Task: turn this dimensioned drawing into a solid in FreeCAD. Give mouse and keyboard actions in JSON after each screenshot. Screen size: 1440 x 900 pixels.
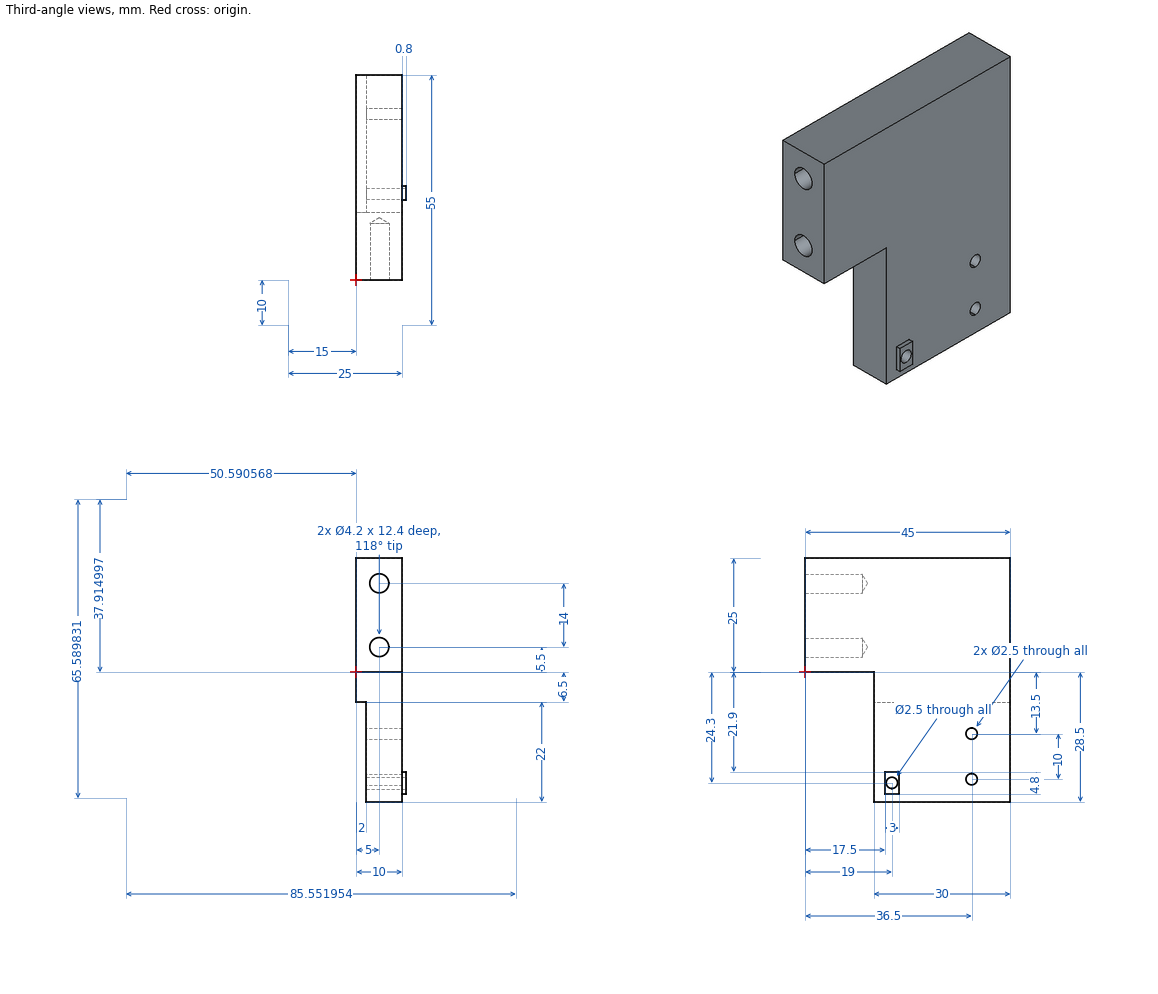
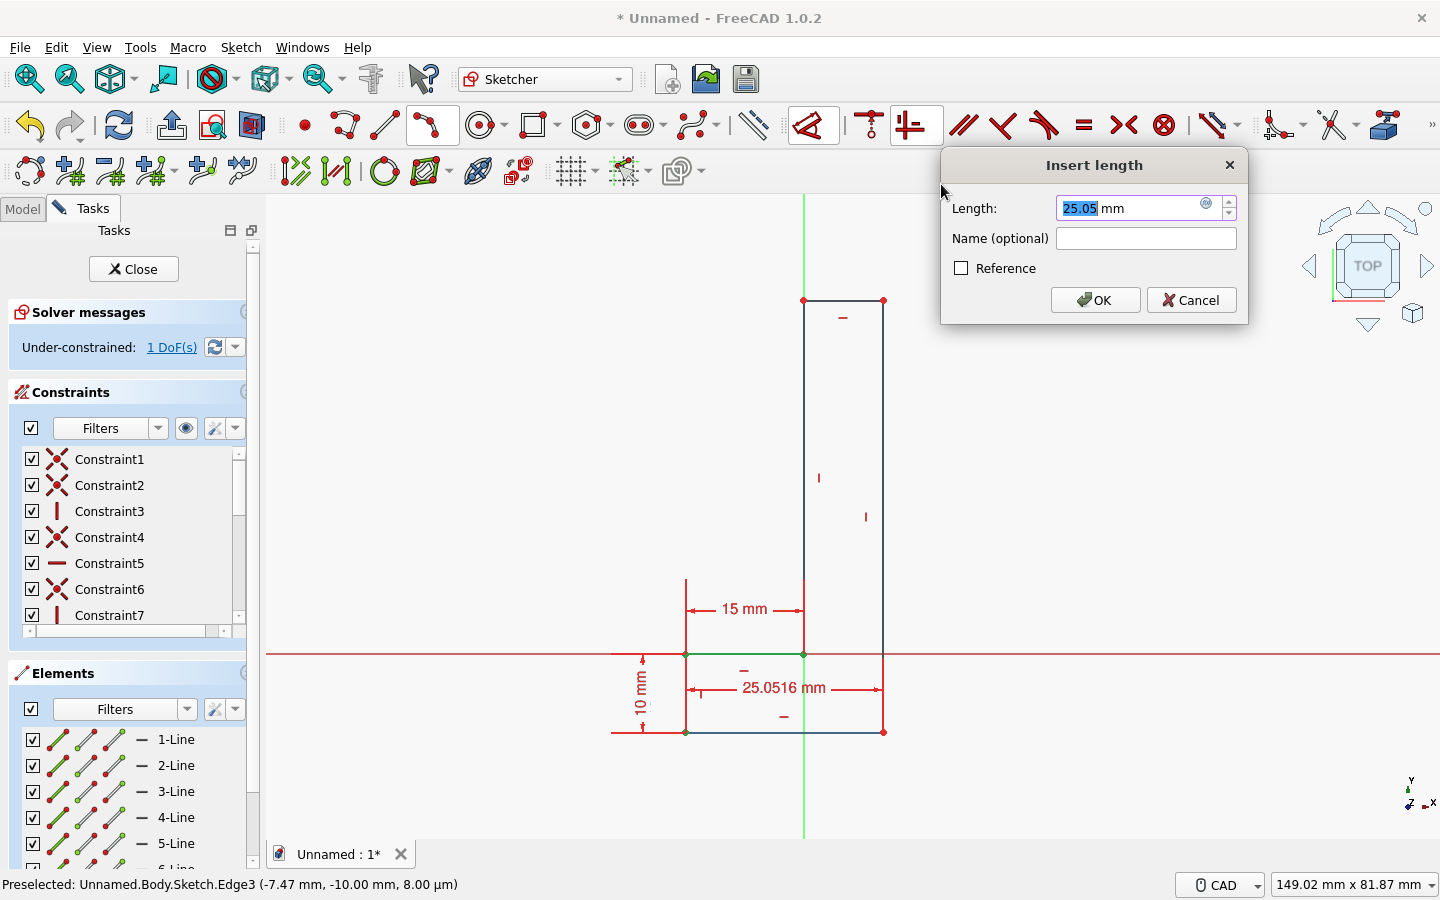
{"action": "type", "text": "25"}
{"action": "key", "text": "Return"}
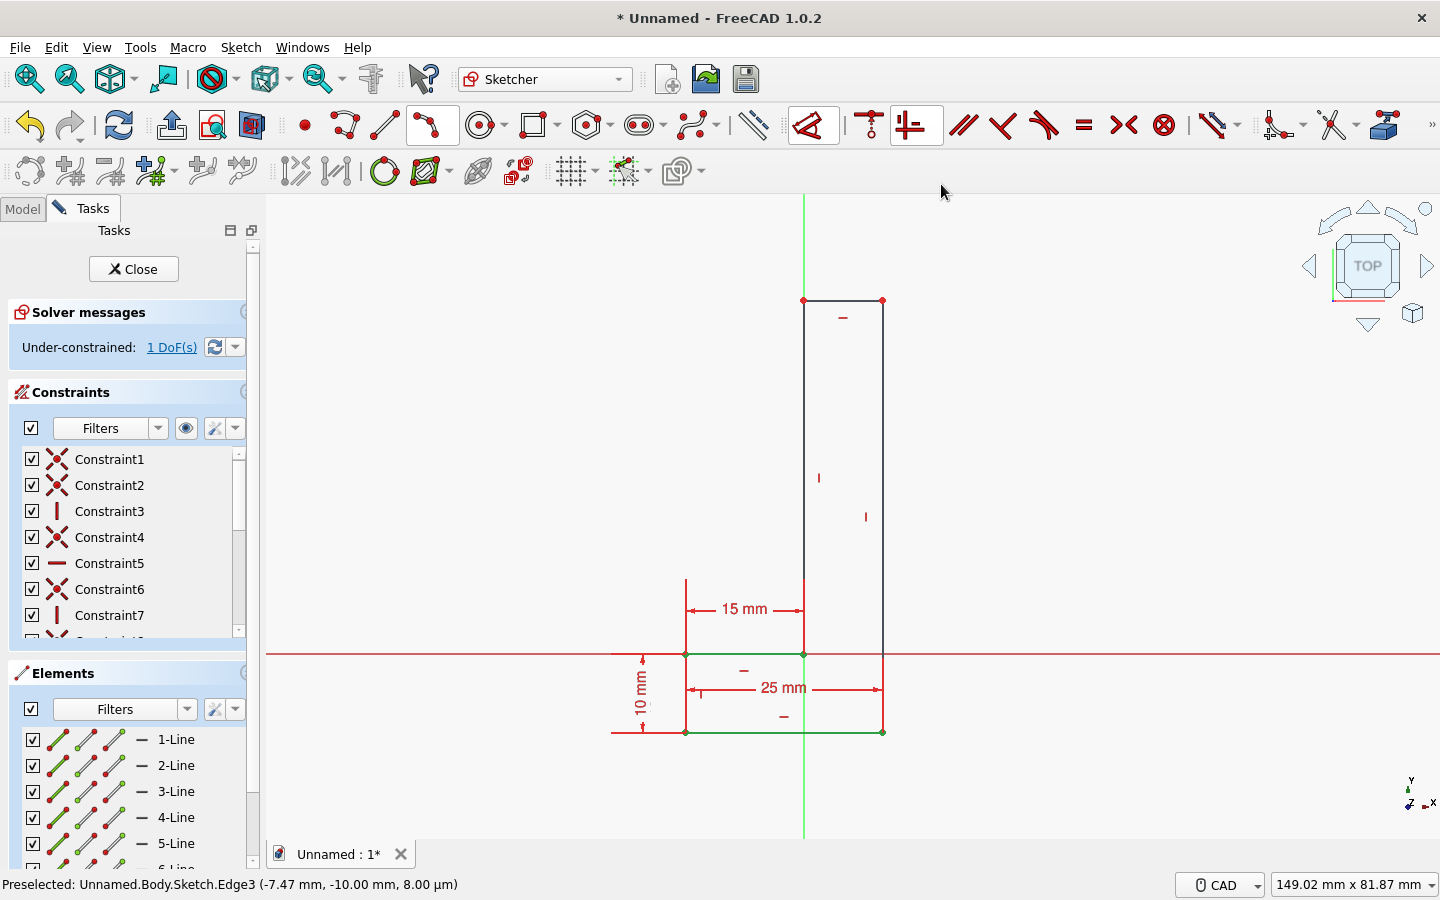
{"action": "left_click", "coordinate": [883, 603]}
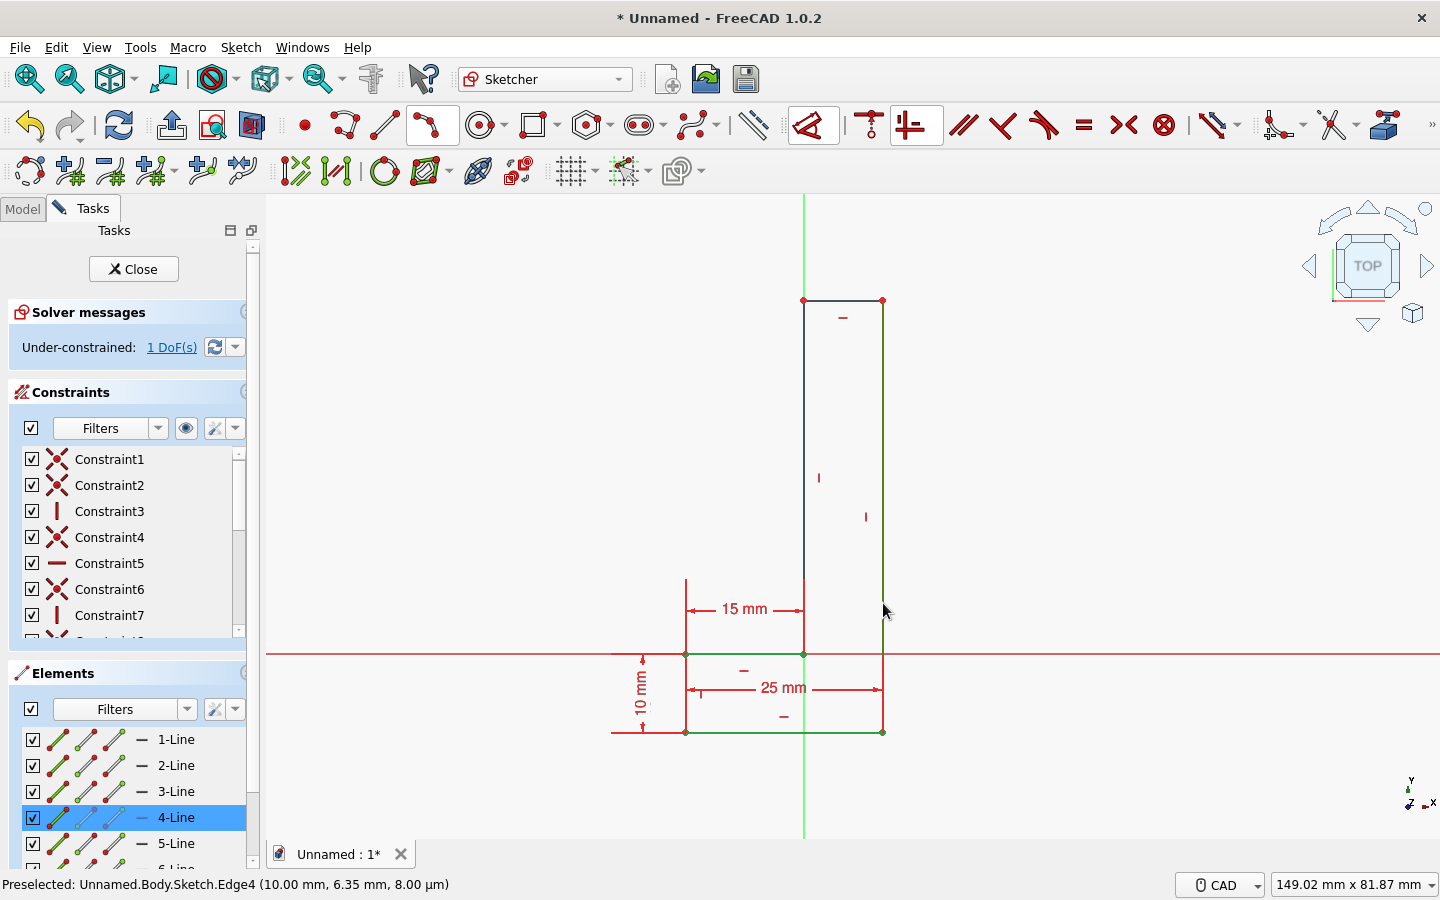
{"action": "key", "text": "i"}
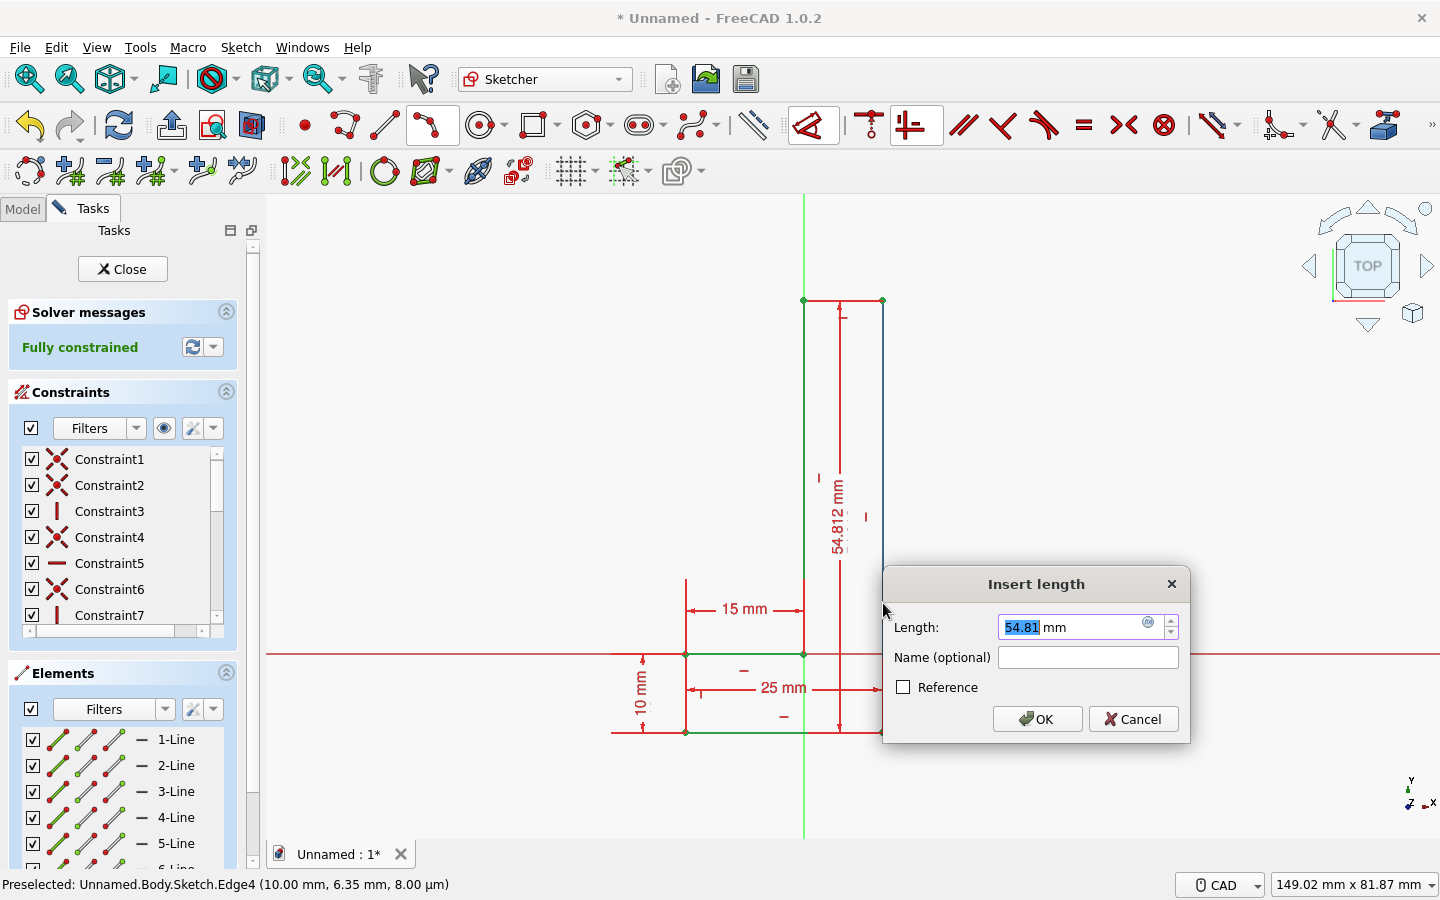
{"action": "type", "text": "55"}
{"action": "key", "text": "Return"}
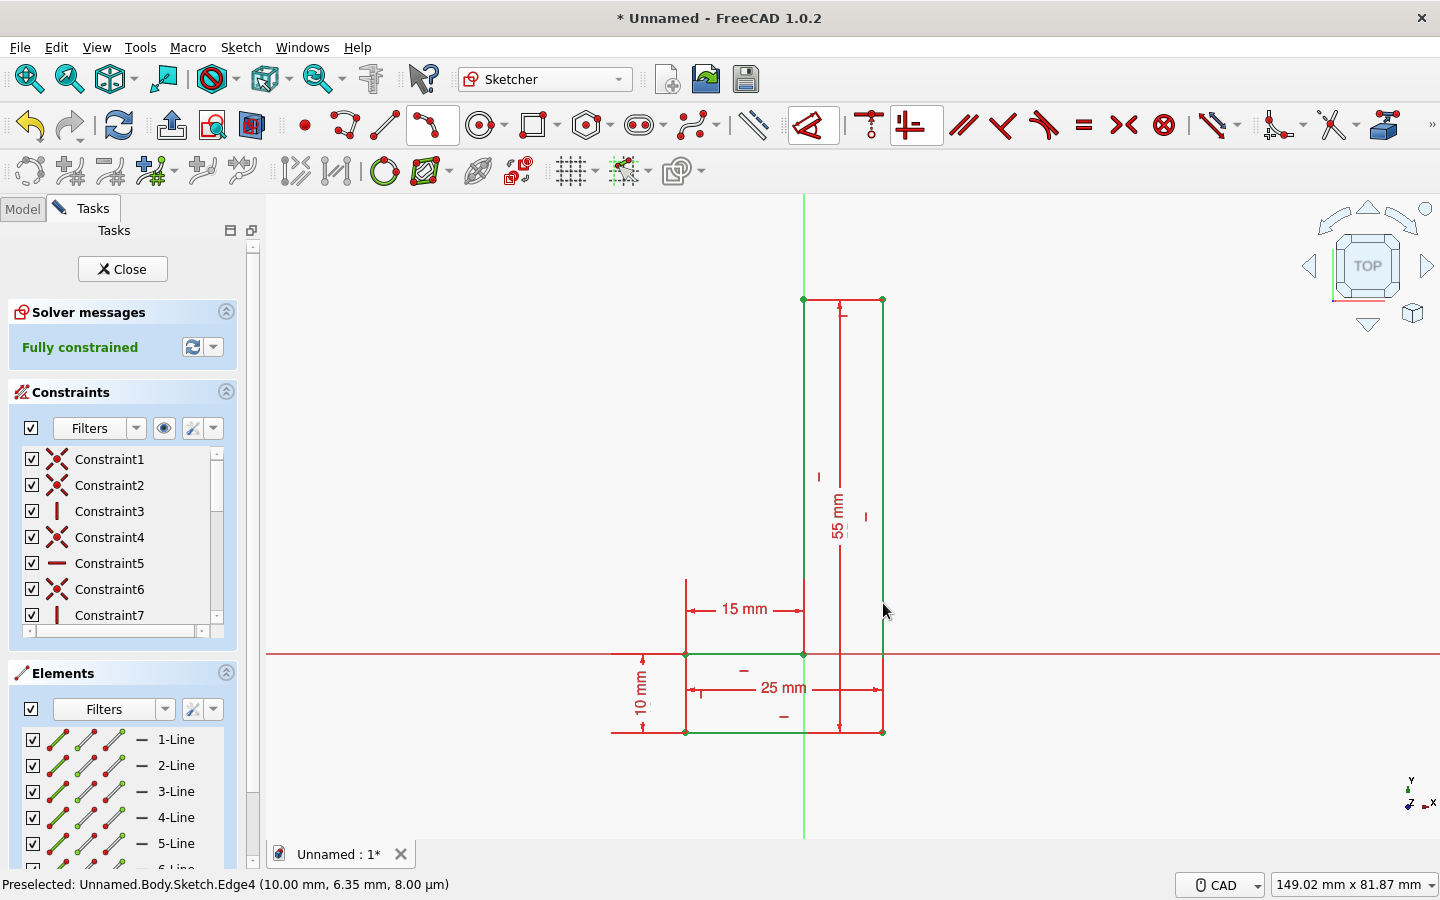
{"action": "left_click", "coordinate": [123, 269]}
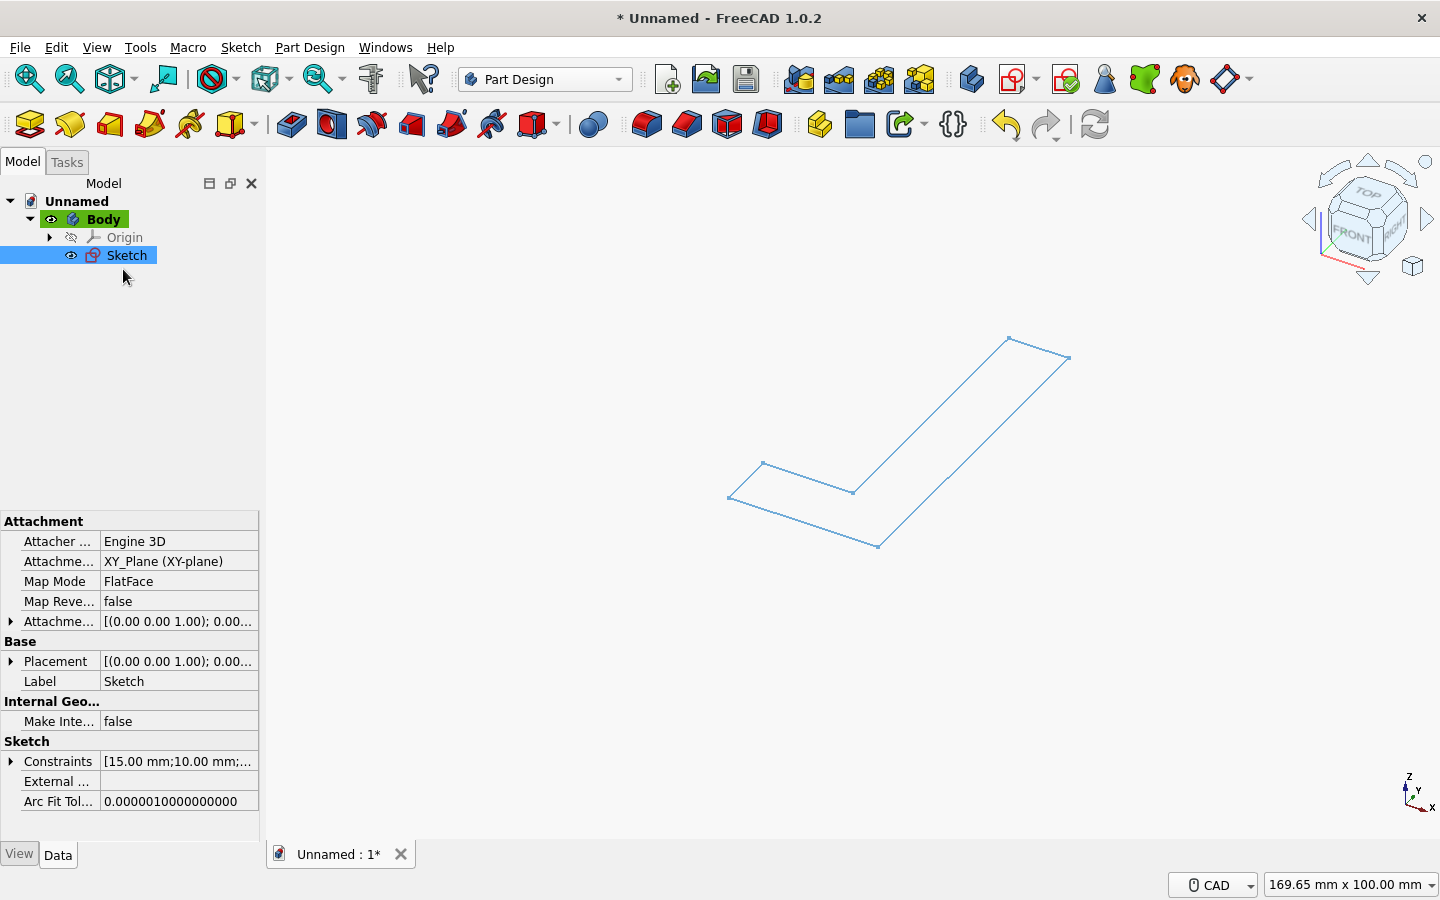
{"action": "left_click", "coordinate": [30, 124]}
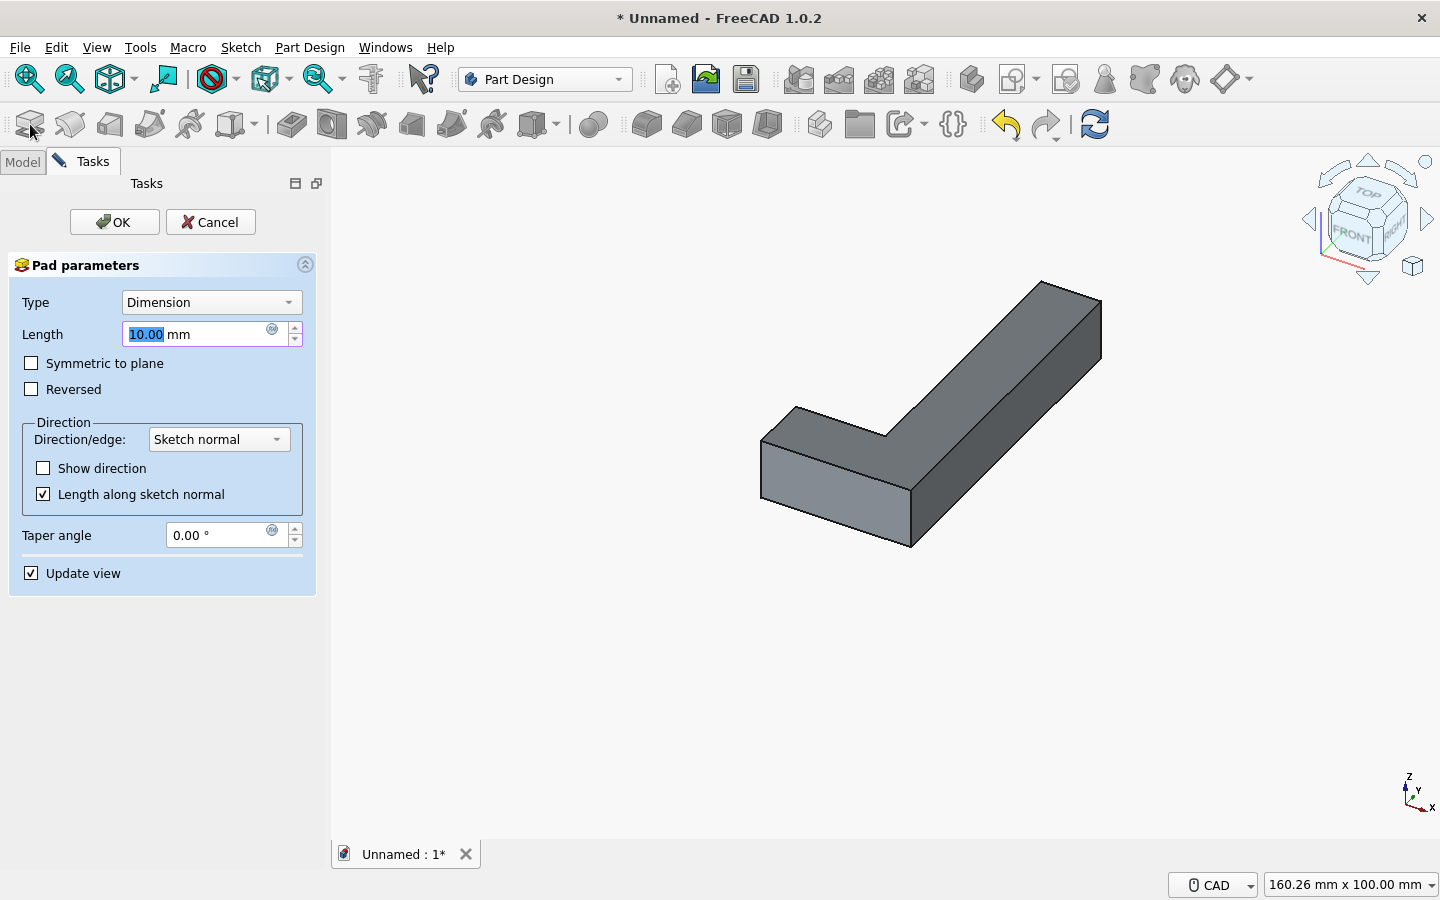
{"action": "type", "text": "25"}
{"action": "key", "text": "Tab"}